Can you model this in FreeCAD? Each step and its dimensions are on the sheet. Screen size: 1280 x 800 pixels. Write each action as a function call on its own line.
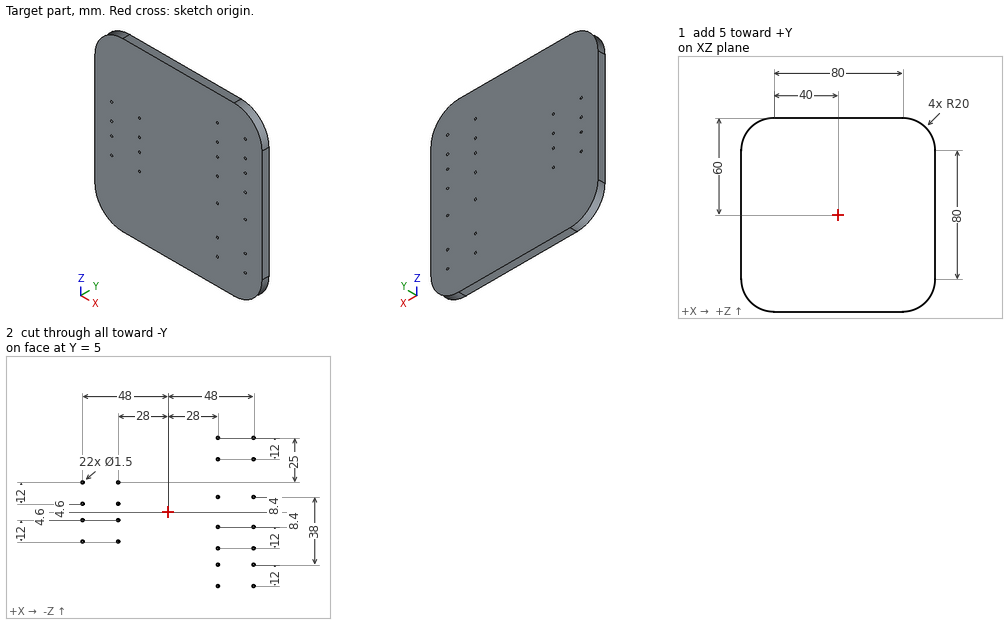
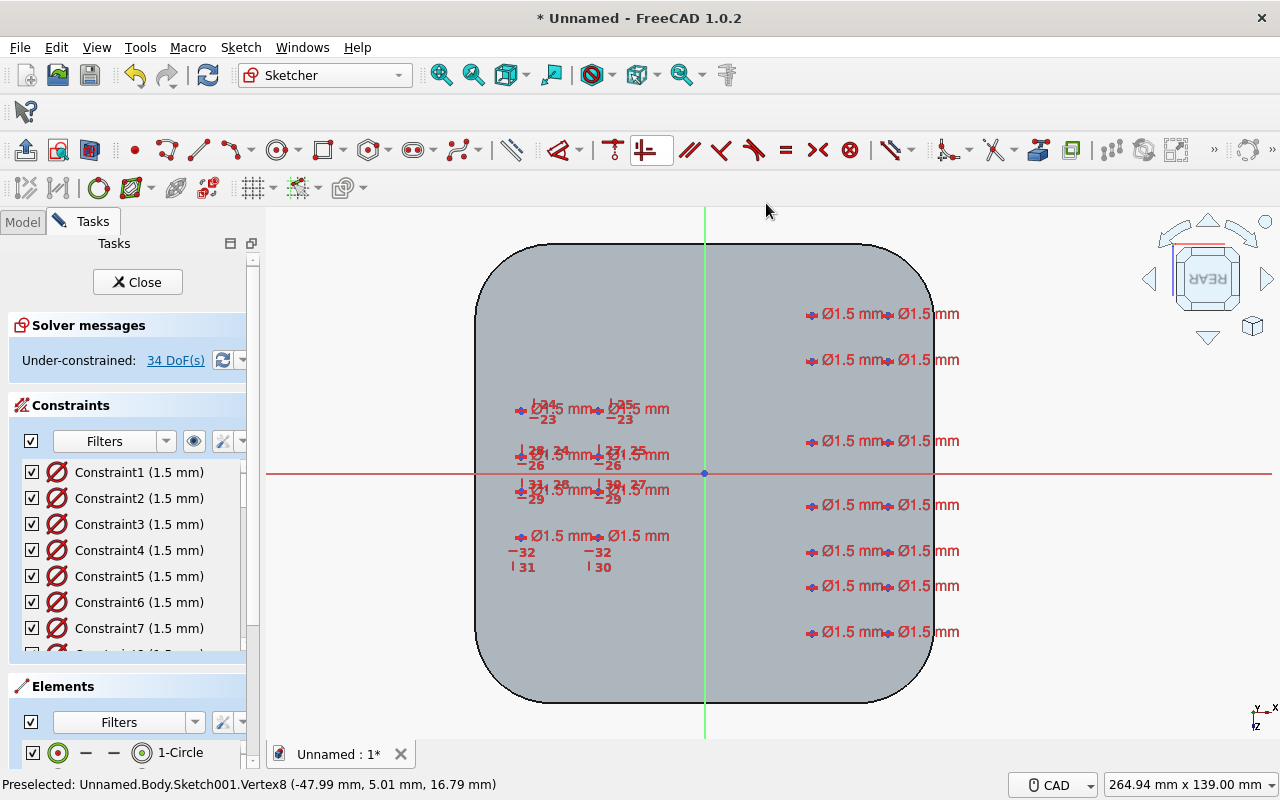
click(812, 316)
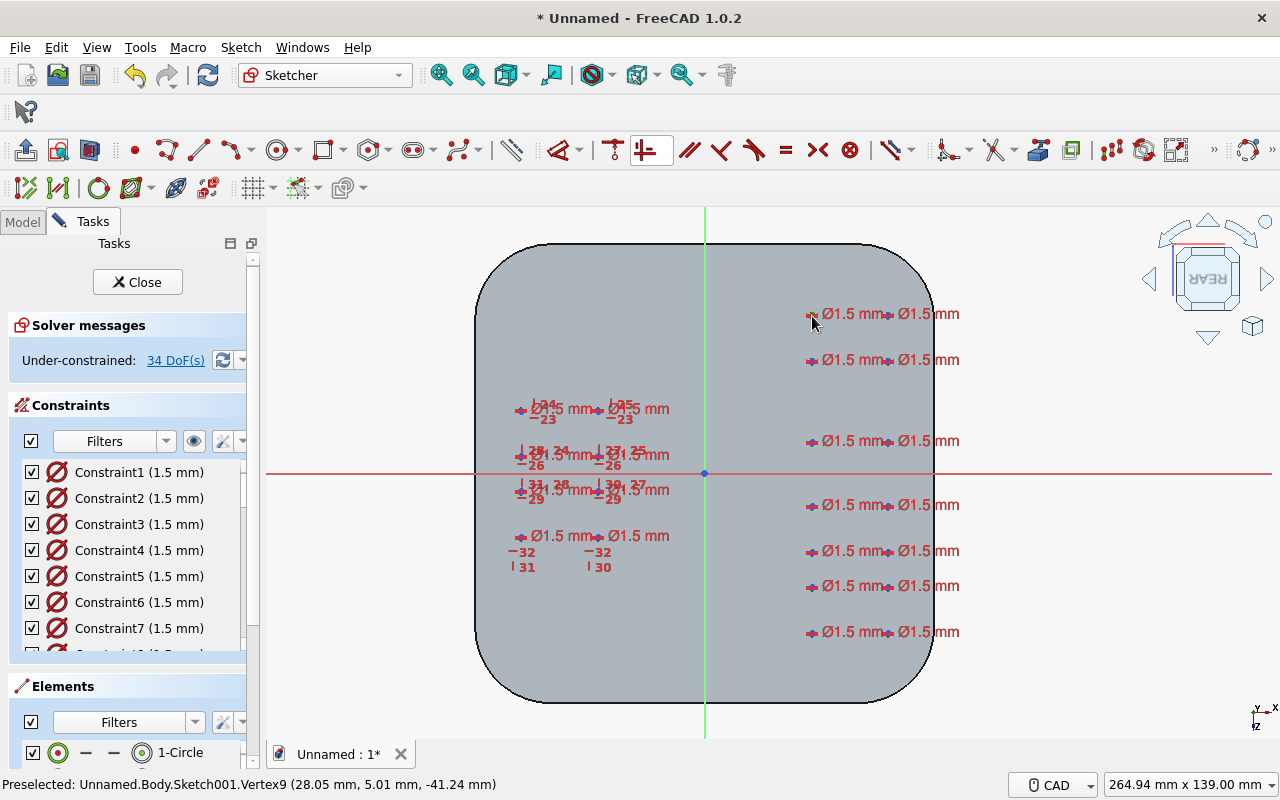
click(888, 316)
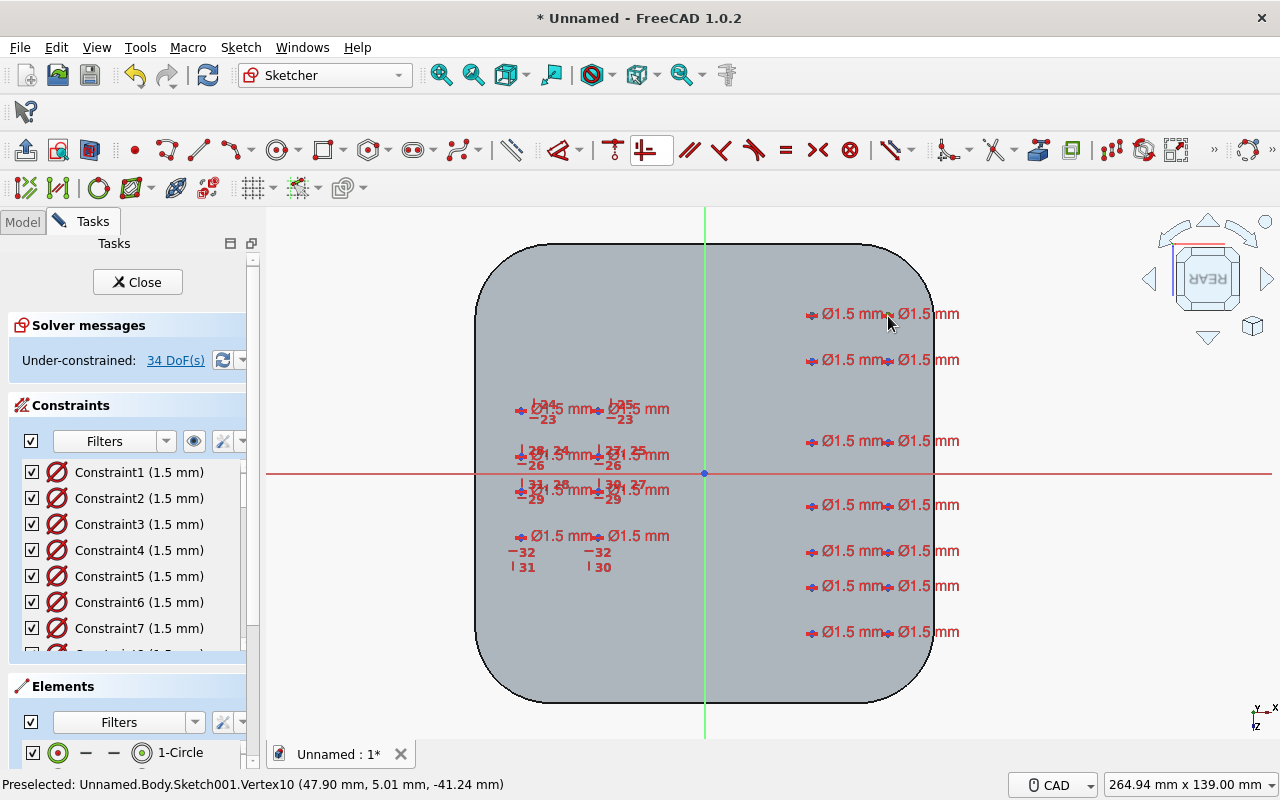
click(668, 150)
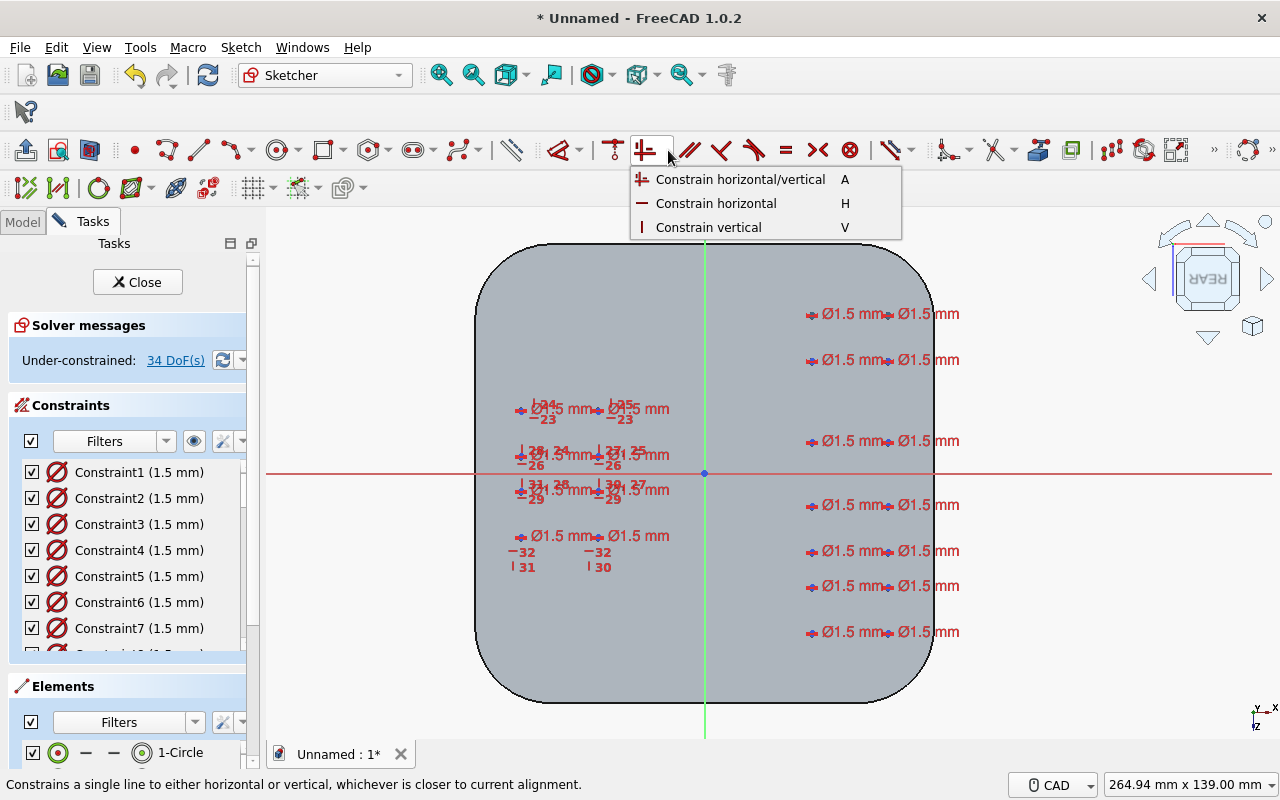
click(766, 203)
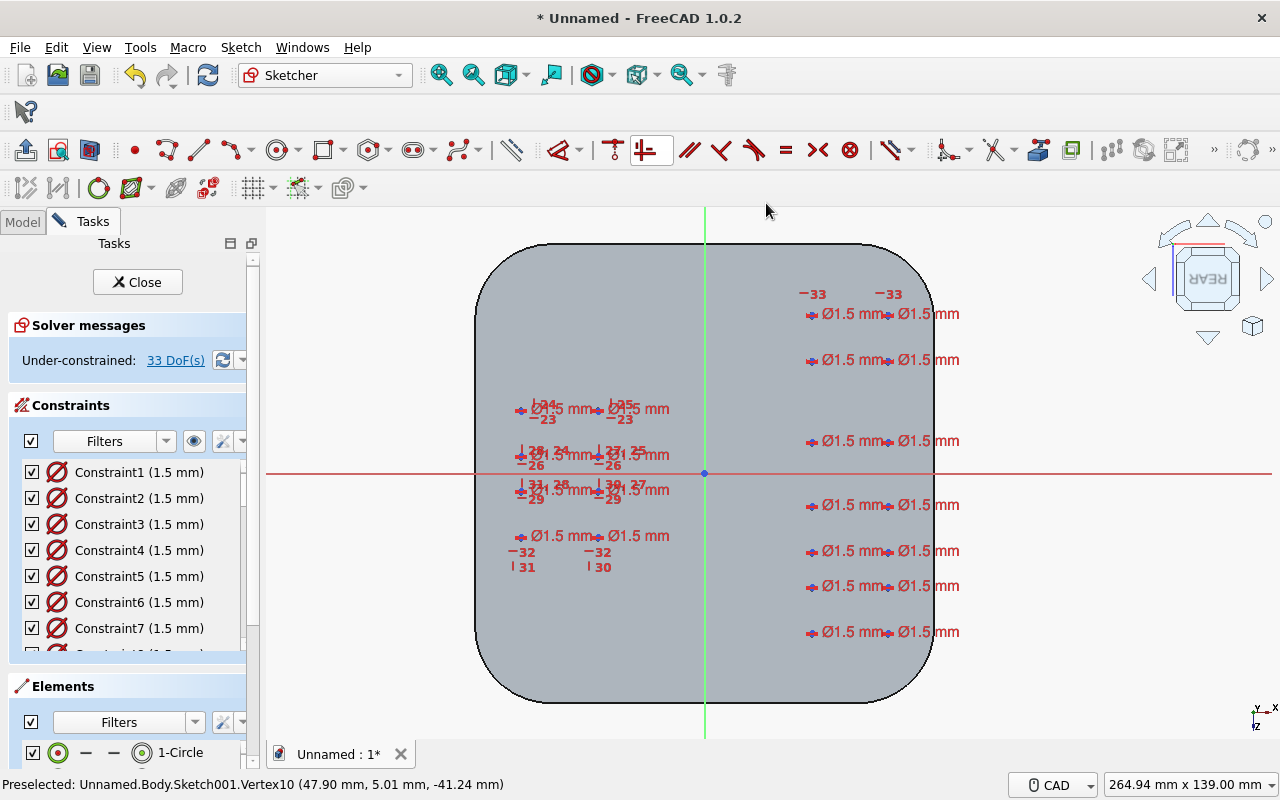
click(812, 316)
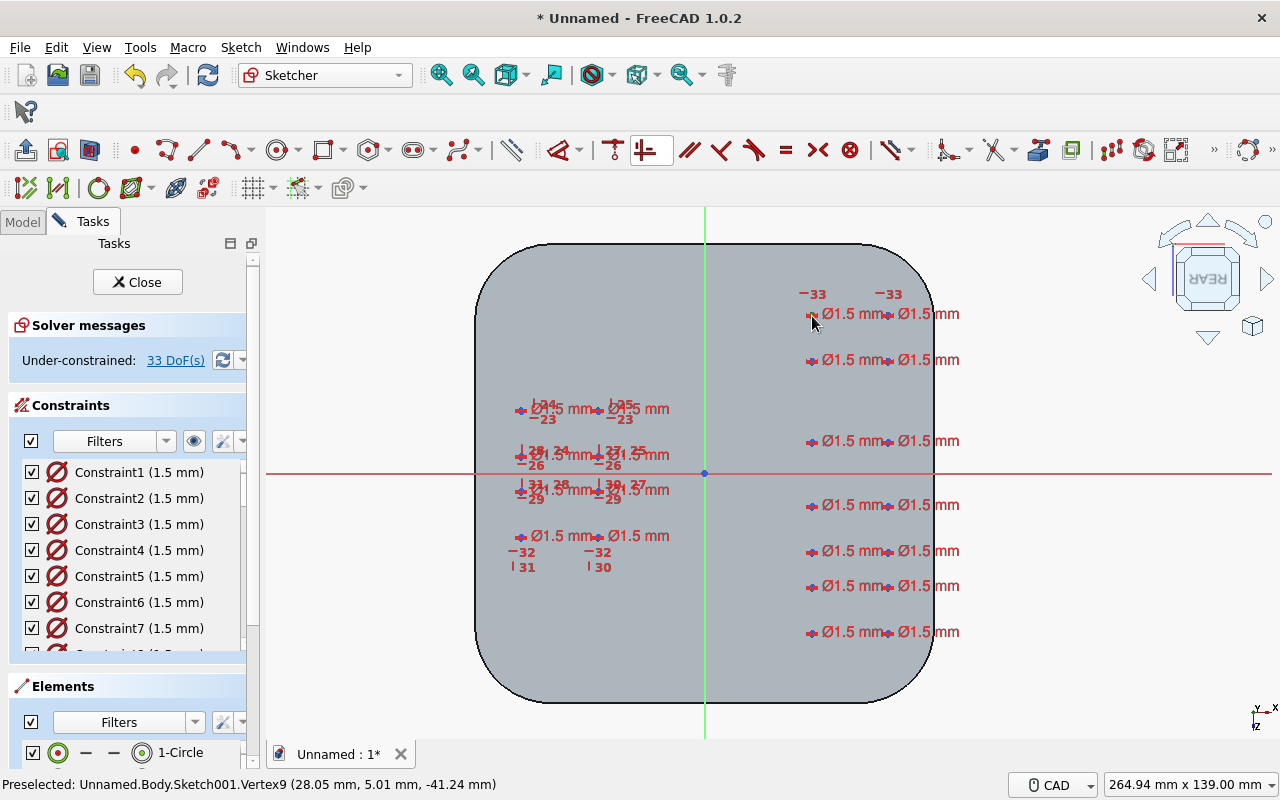
click(812, 362)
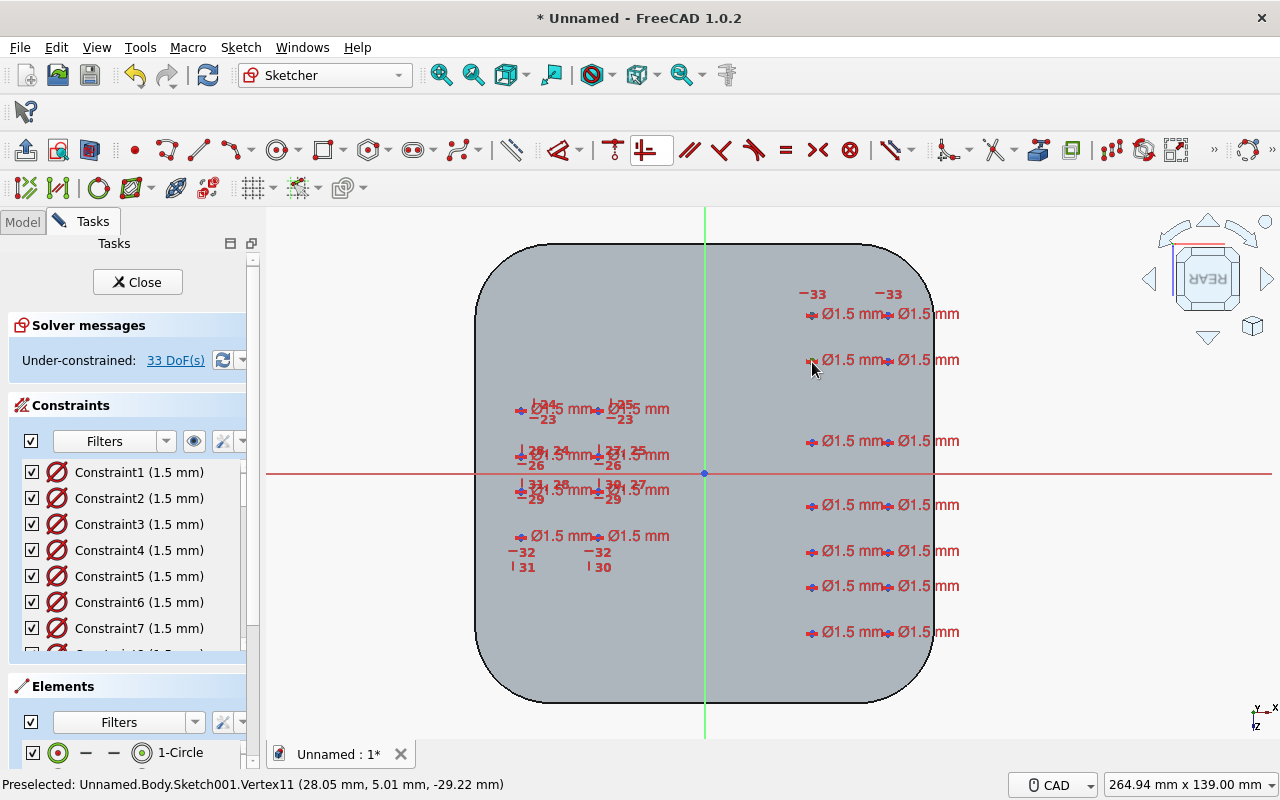
key(v)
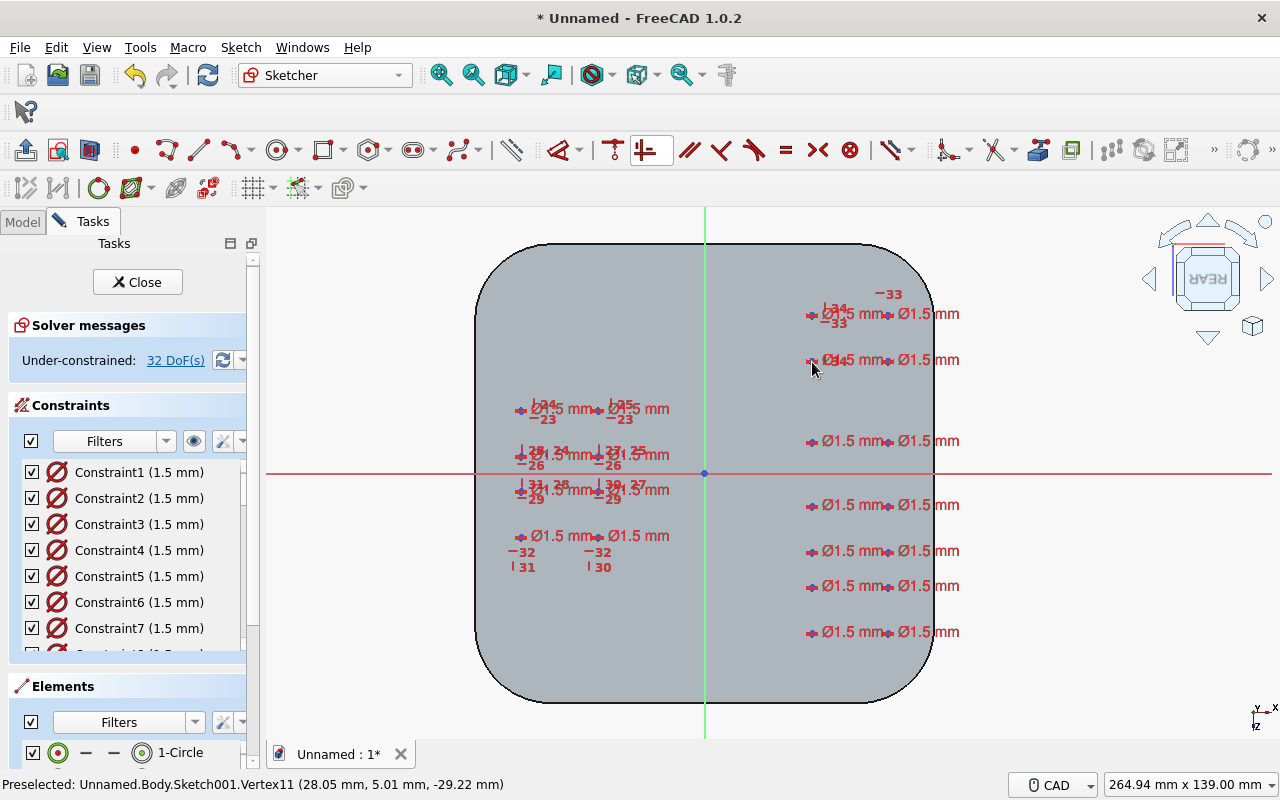
click(888, 316)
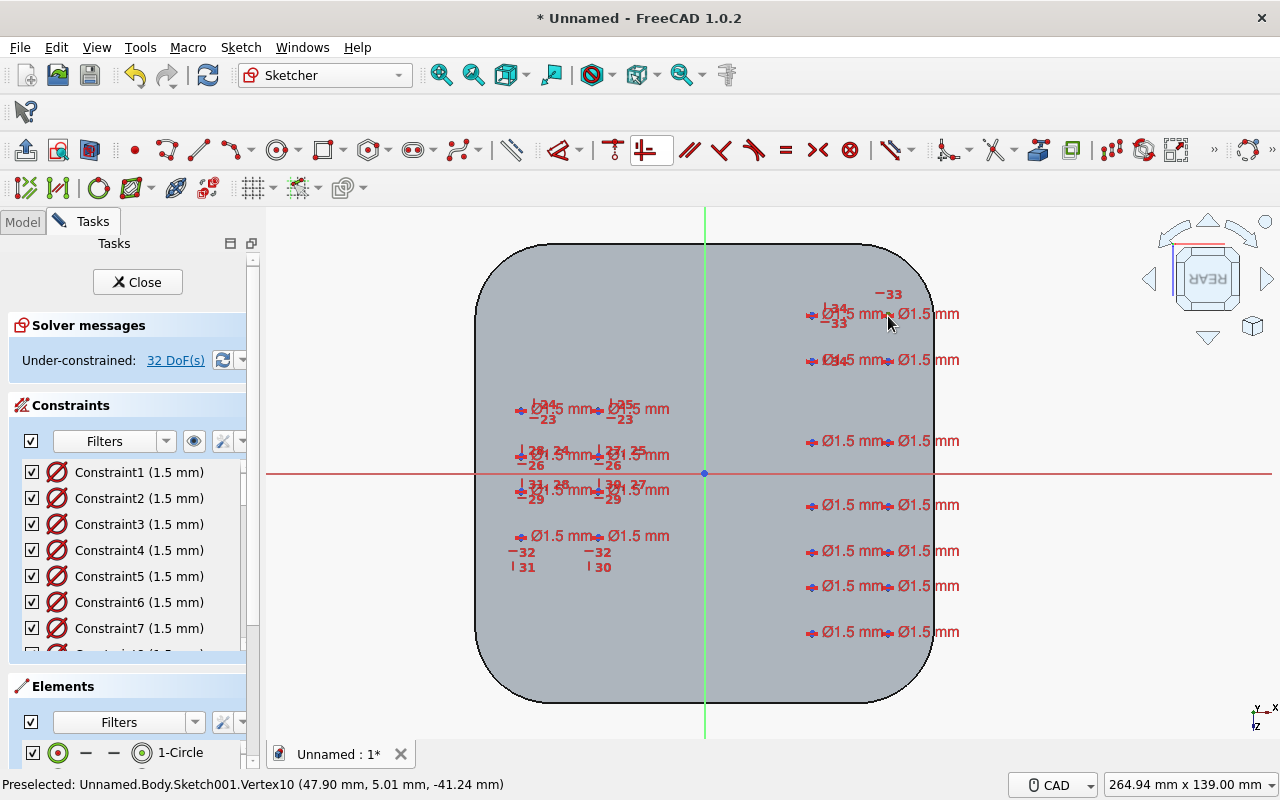
click(888, 362)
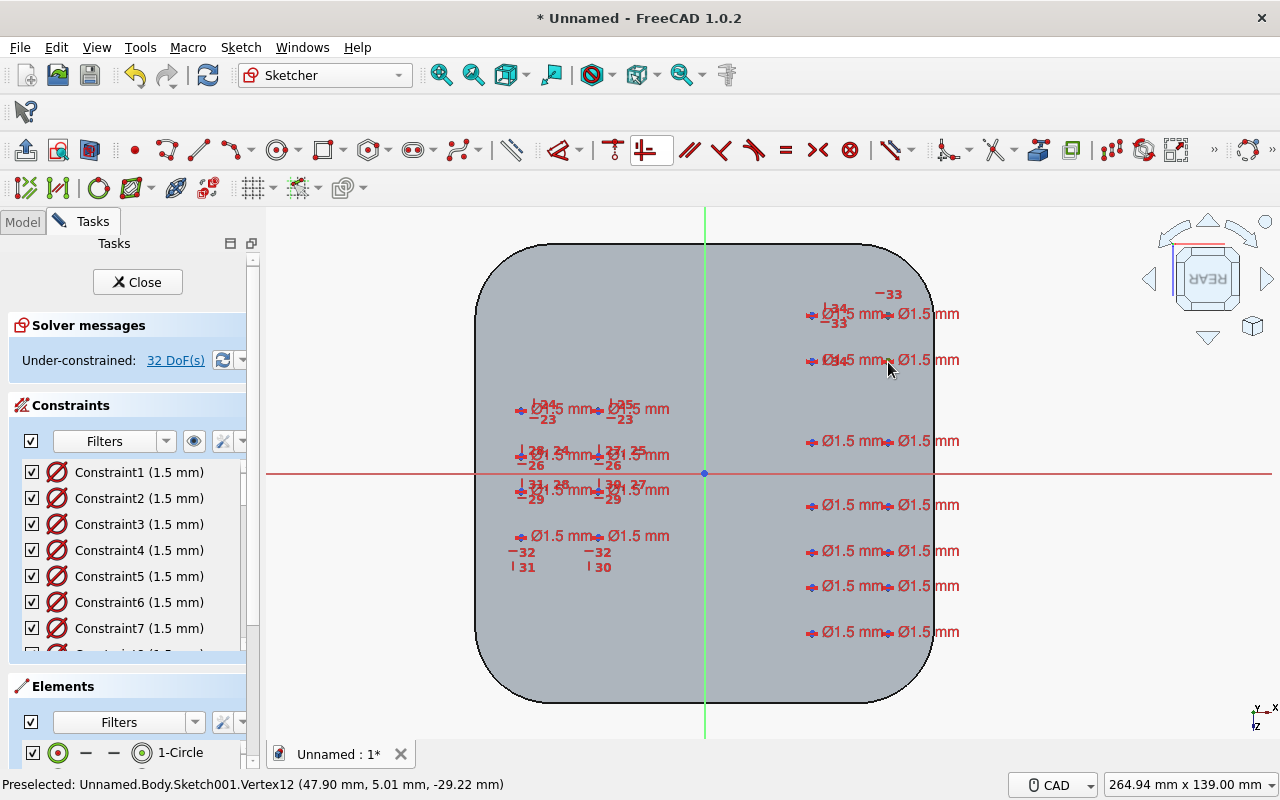
key(v)